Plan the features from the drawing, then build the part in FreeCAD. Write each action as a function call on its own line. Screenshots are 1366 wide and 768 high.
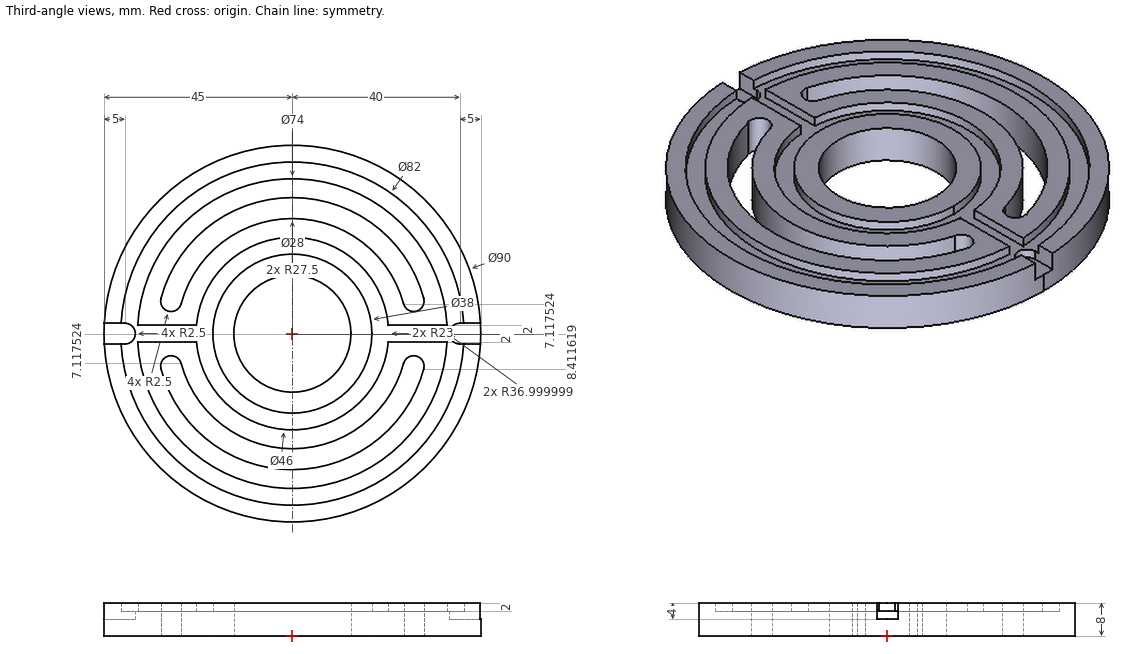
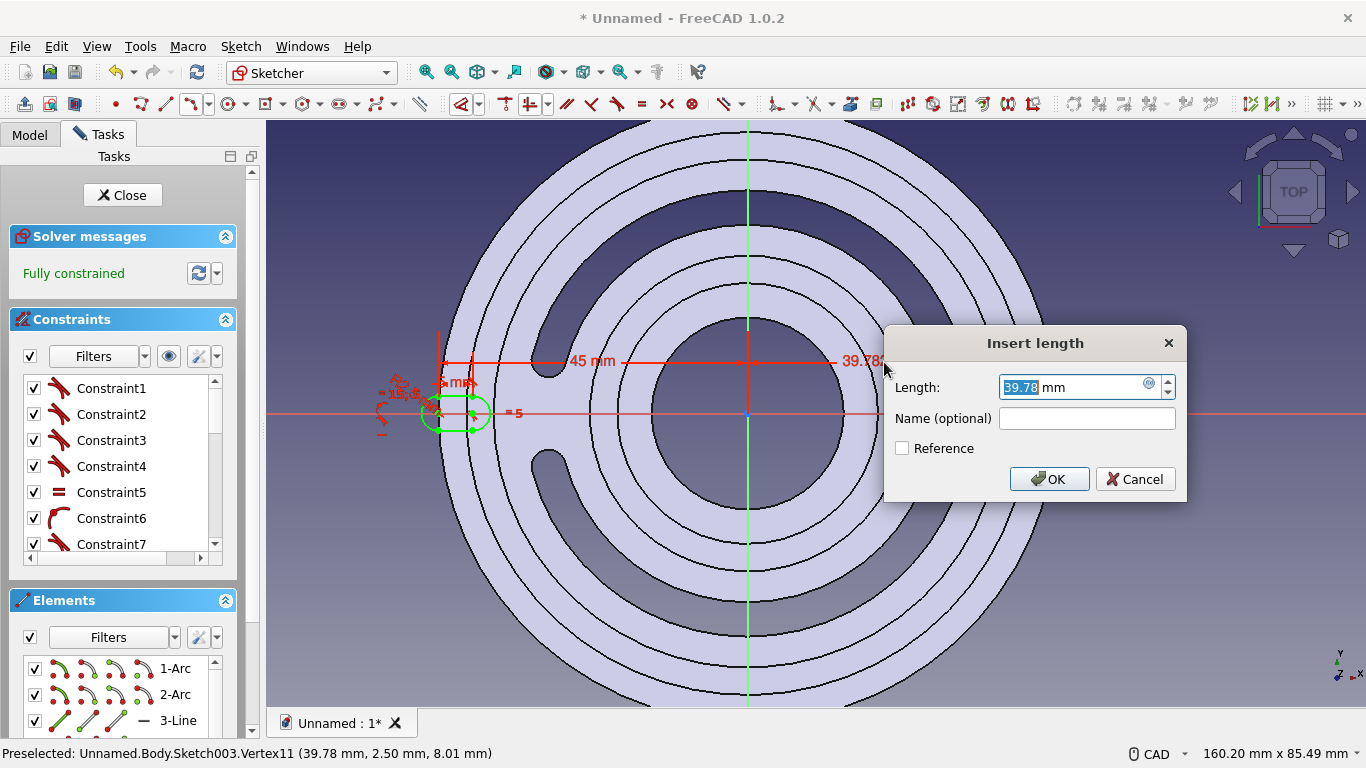
text(40)
key(Return)
key(Escape)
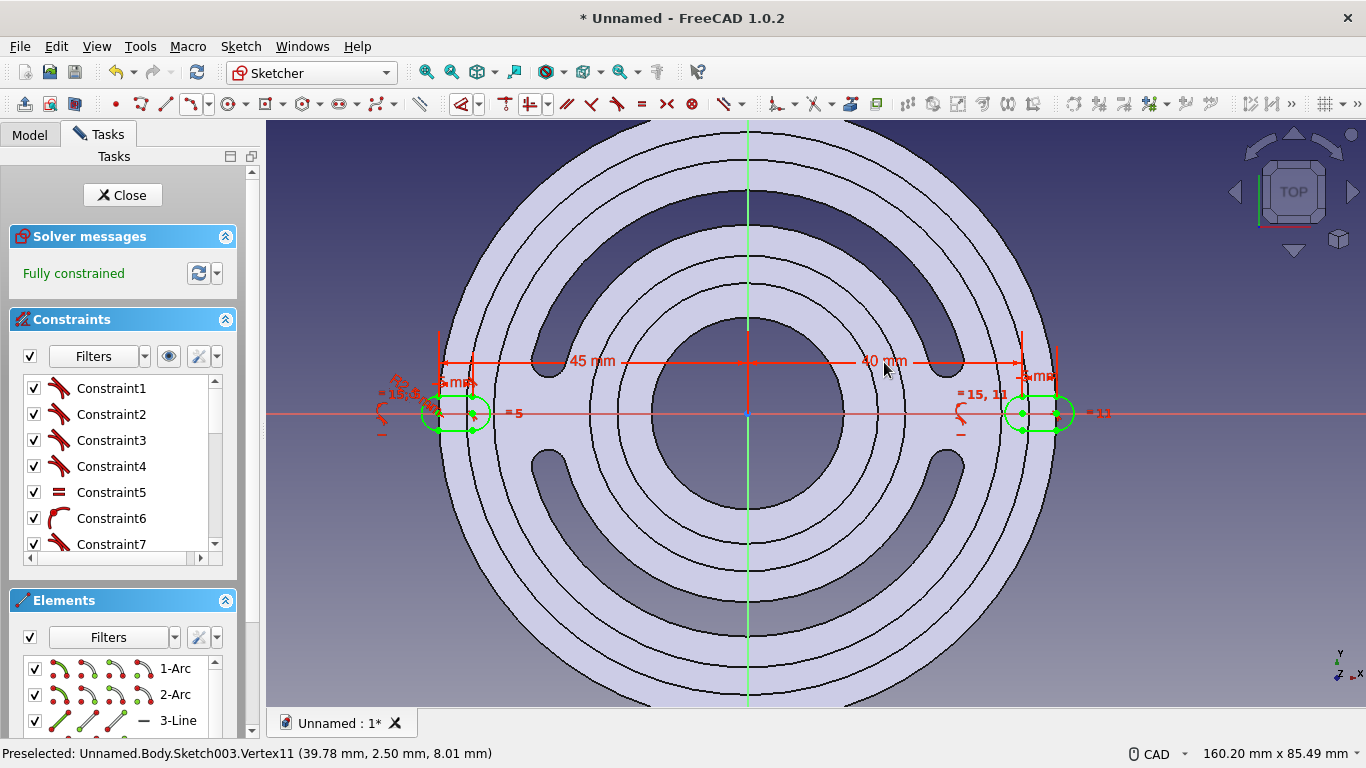
click(123, 195)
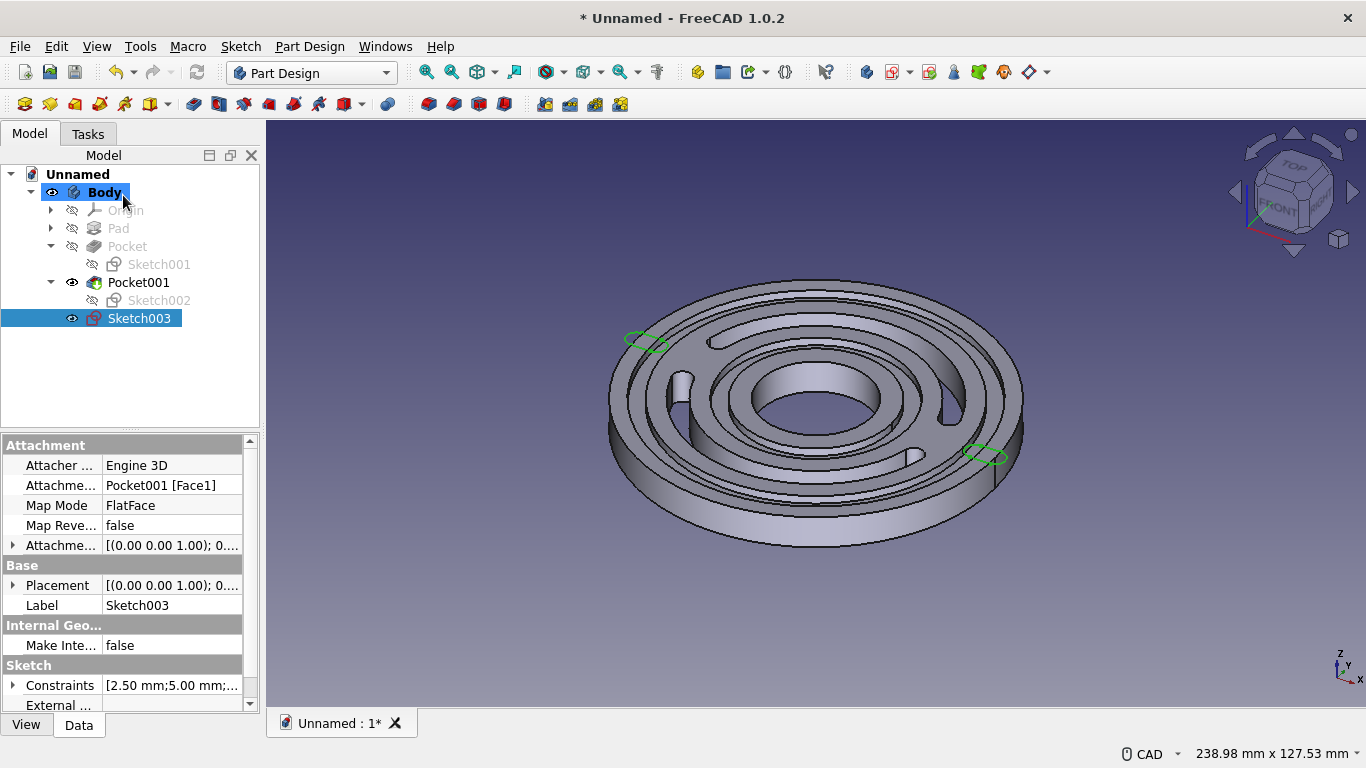
click(194, 104)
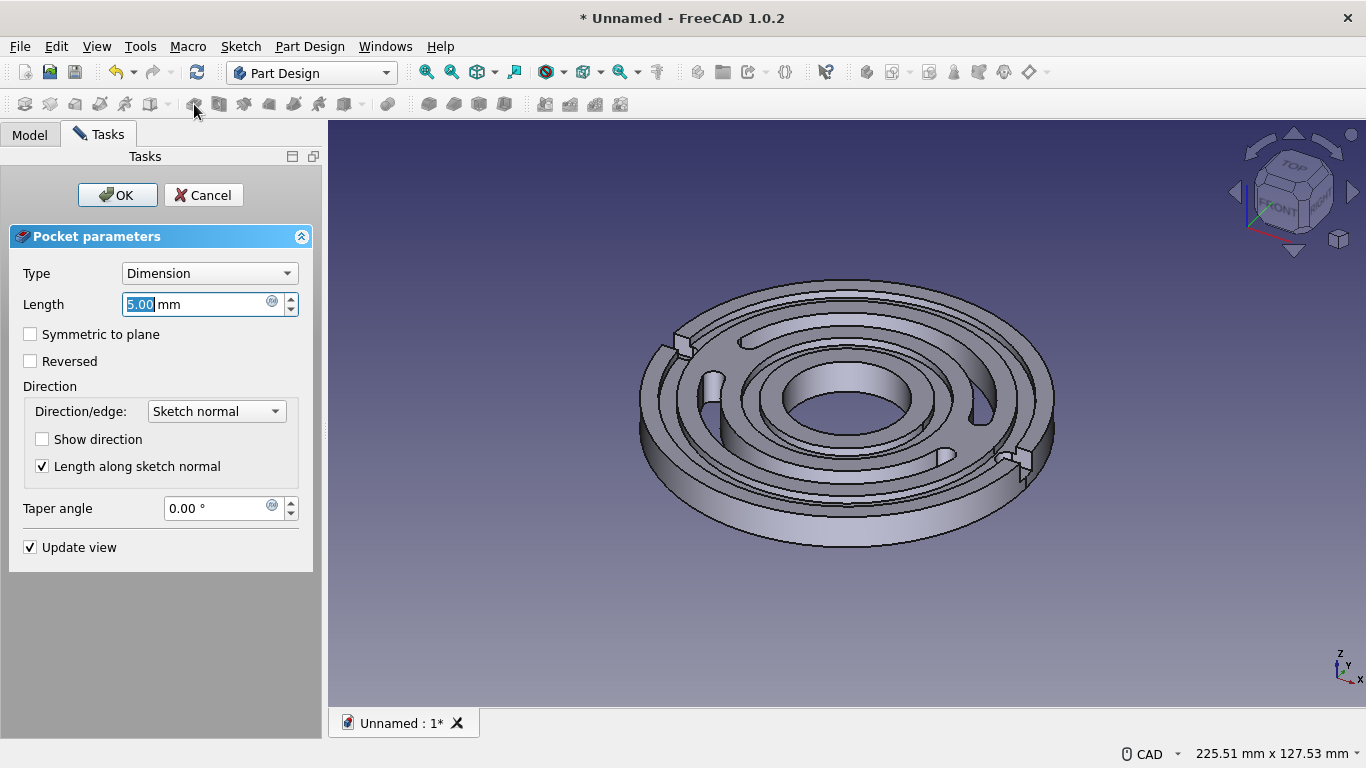
text(4)
key(Tab)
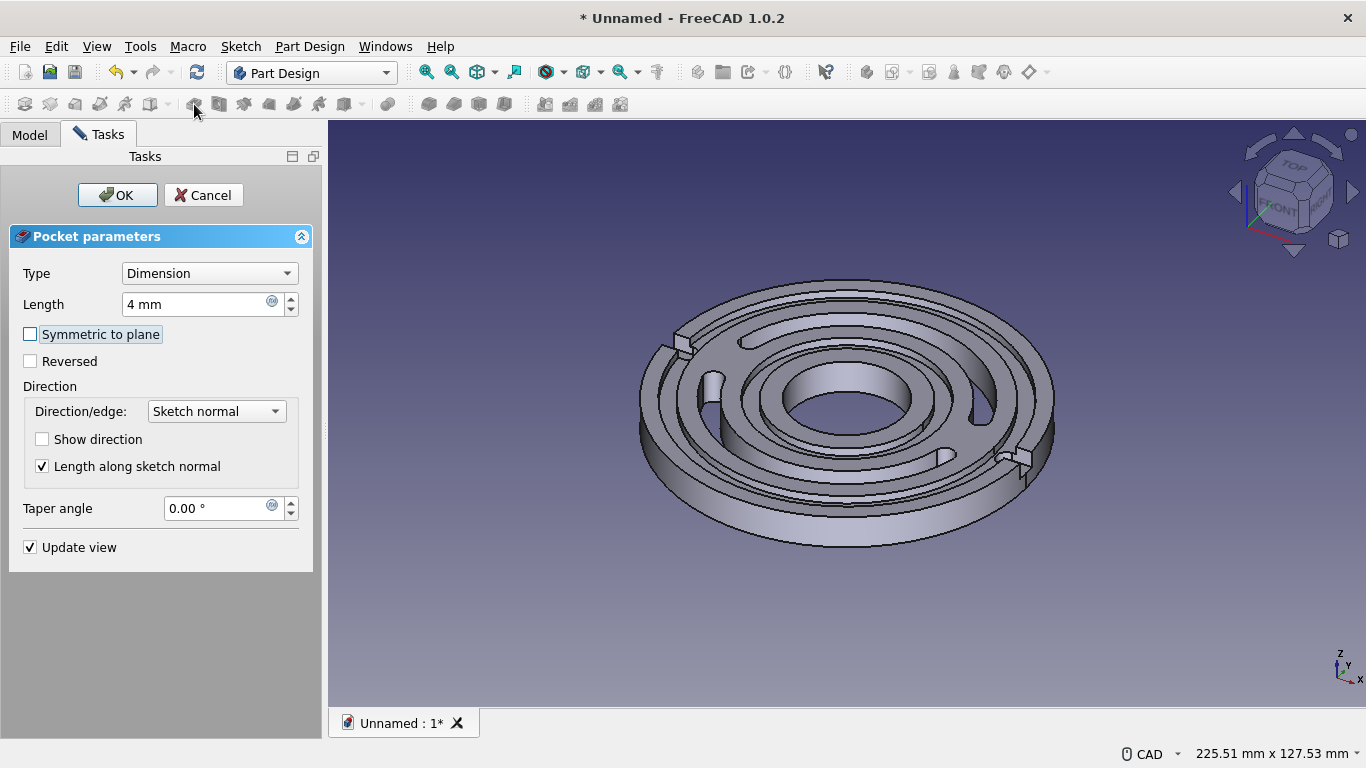
click(118, 195)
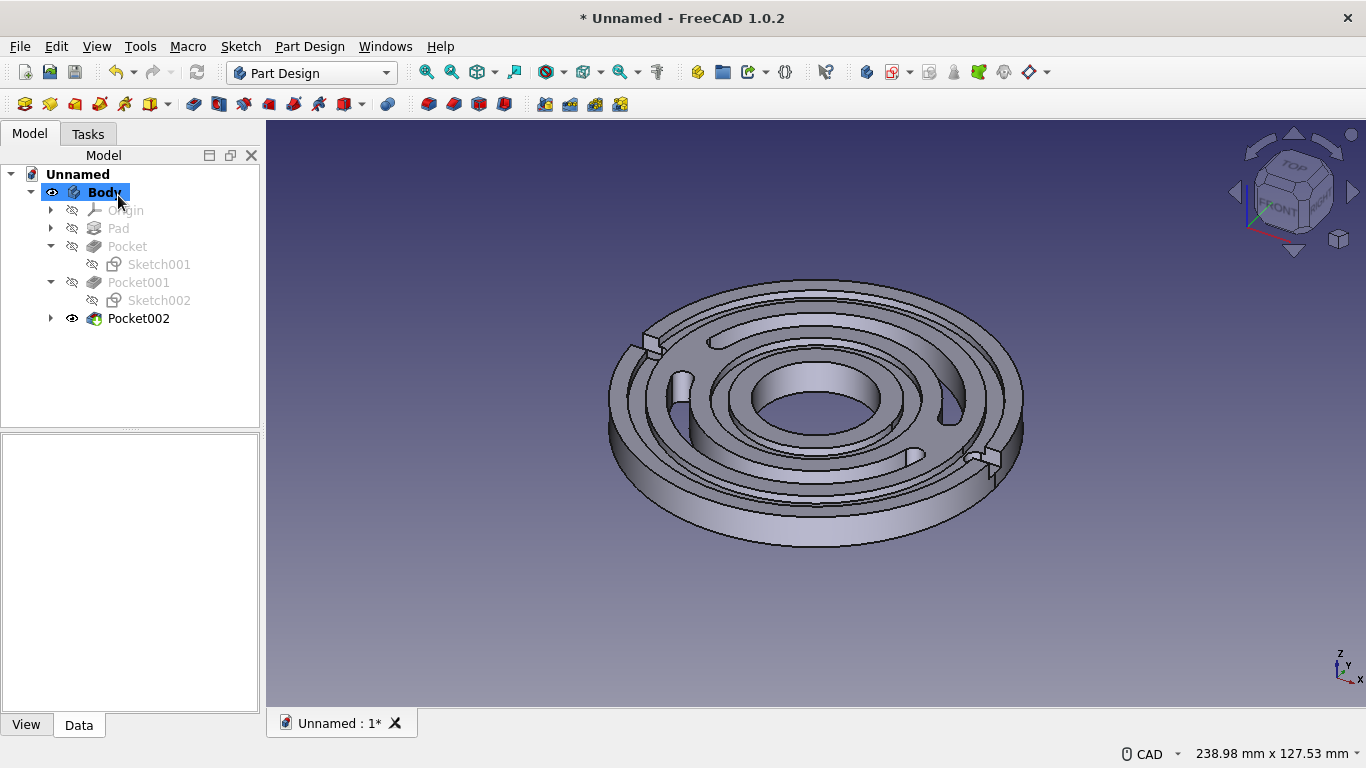
click(942, 439)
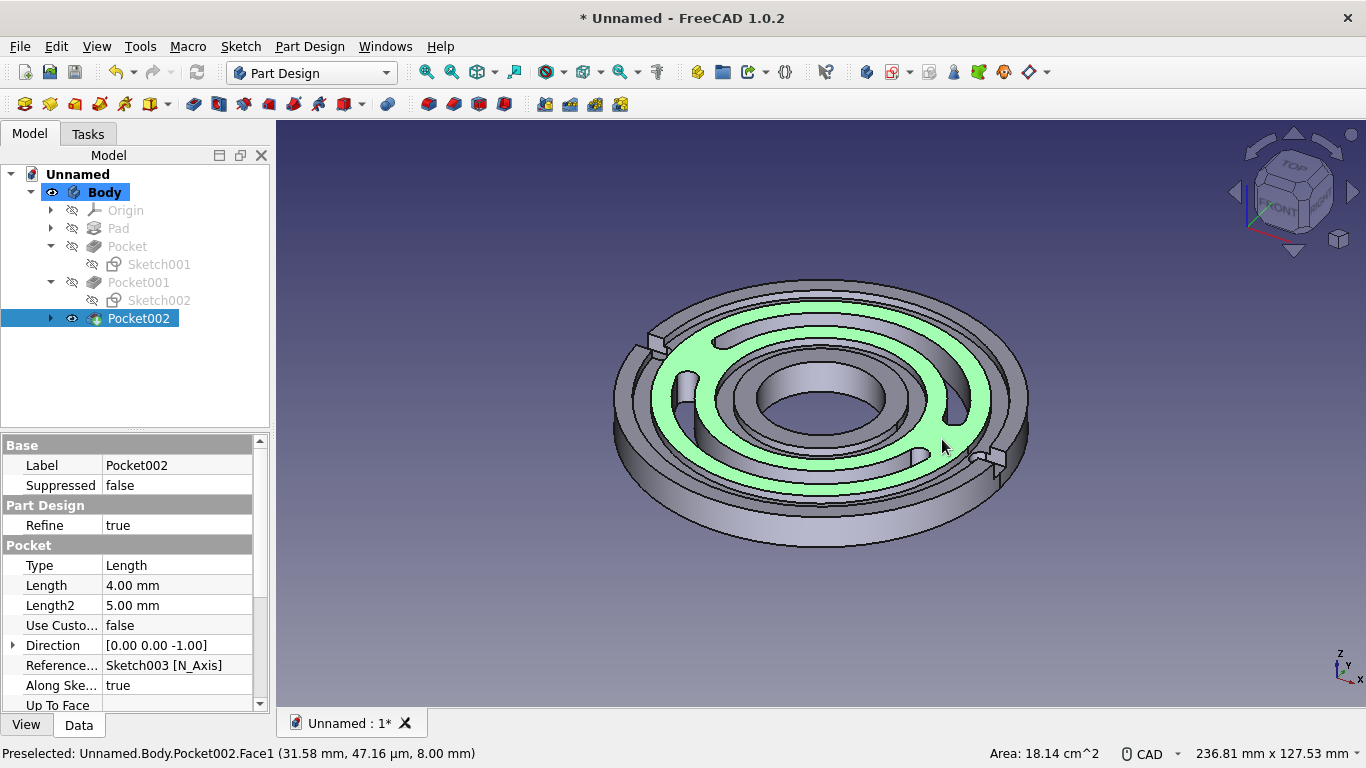
click(892, 72)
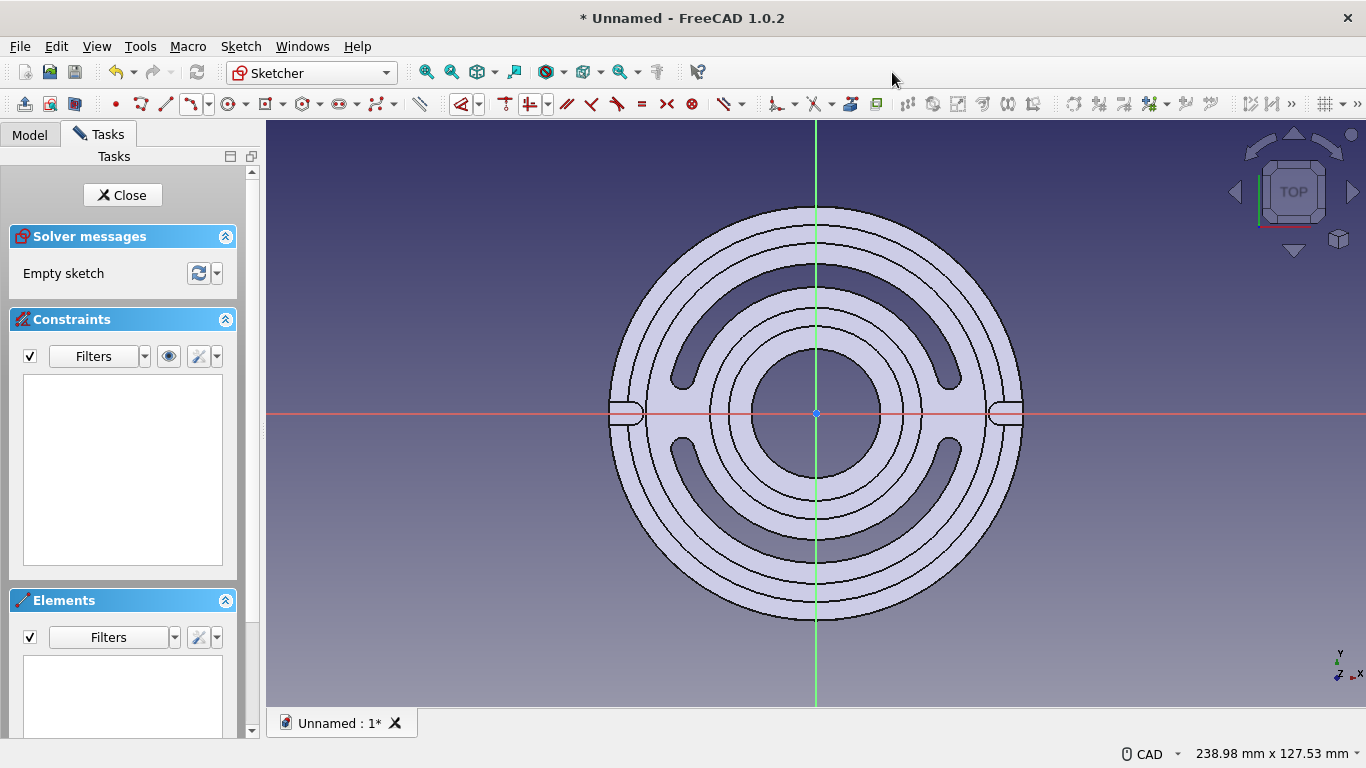
scroll(899, 414, up, 3)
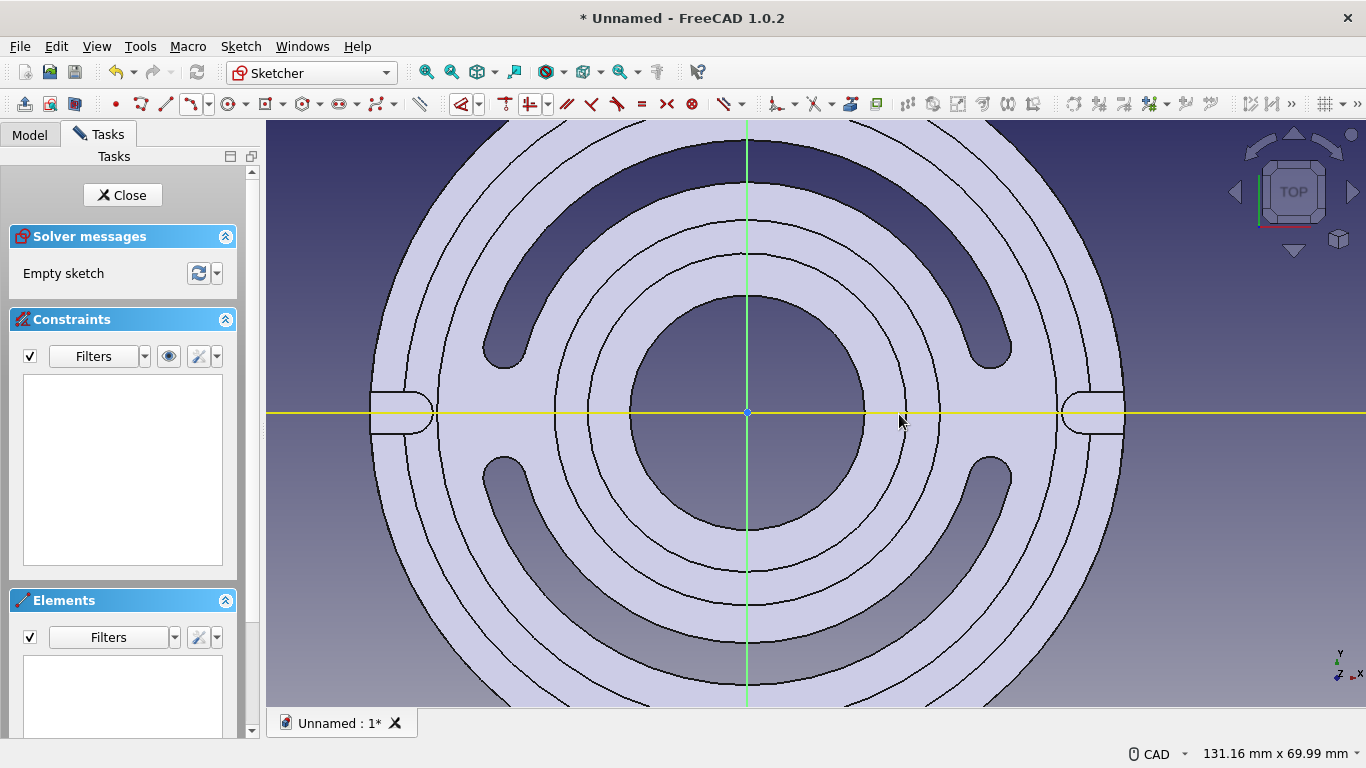
key(g)
key(l)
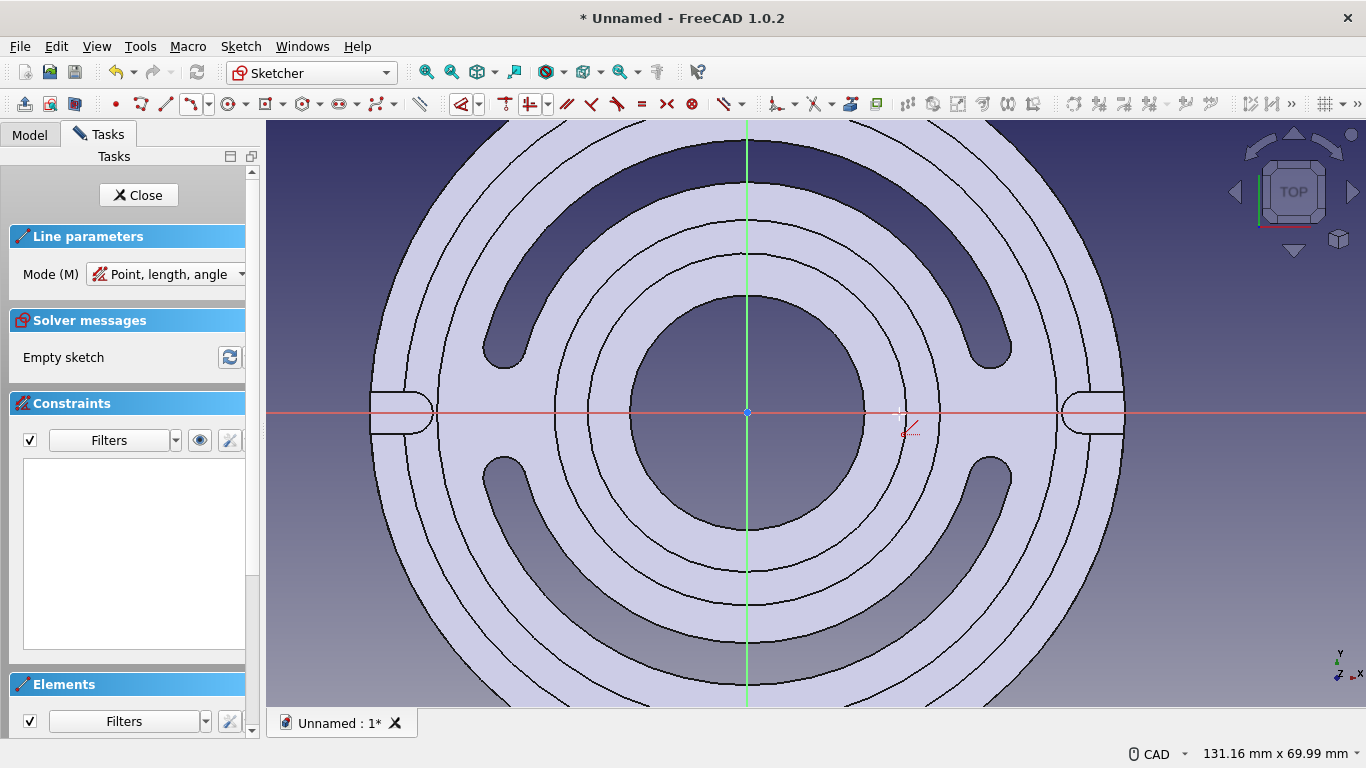
click(939, 429)
click(1057, 429)